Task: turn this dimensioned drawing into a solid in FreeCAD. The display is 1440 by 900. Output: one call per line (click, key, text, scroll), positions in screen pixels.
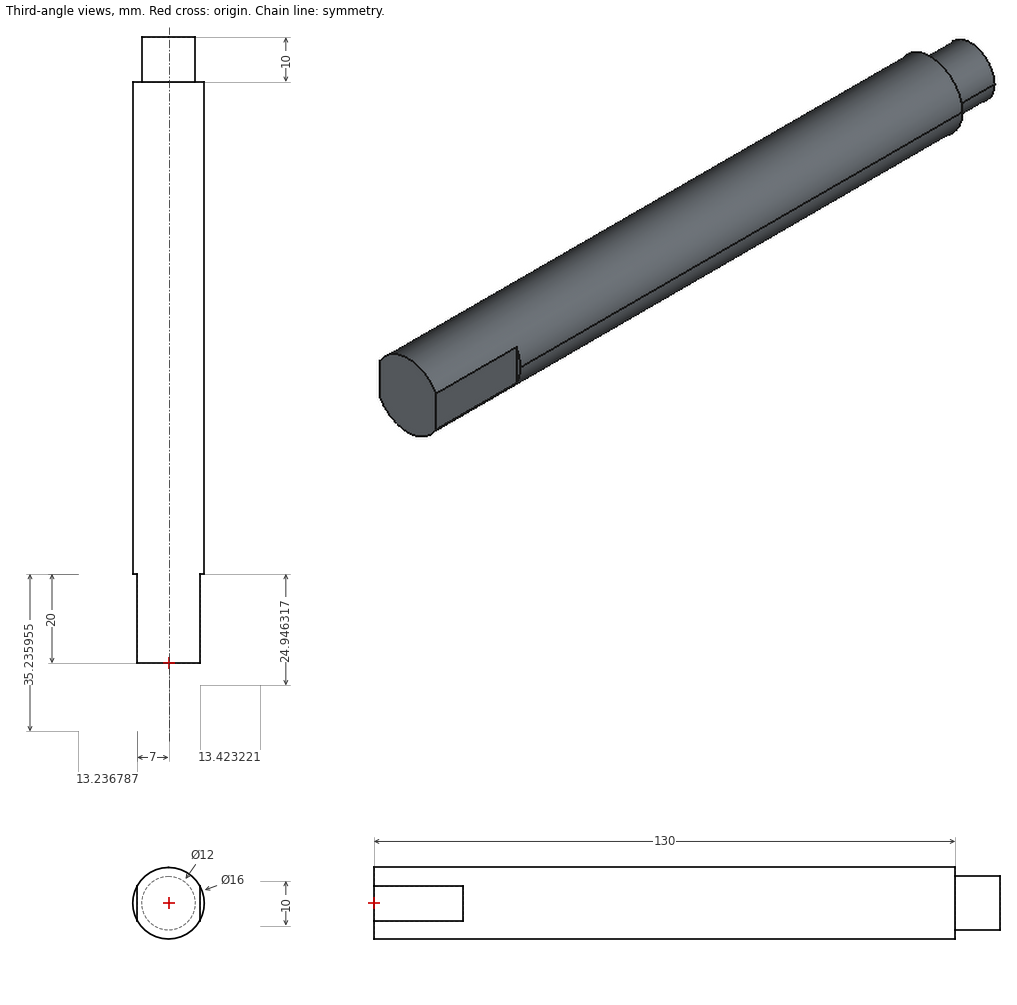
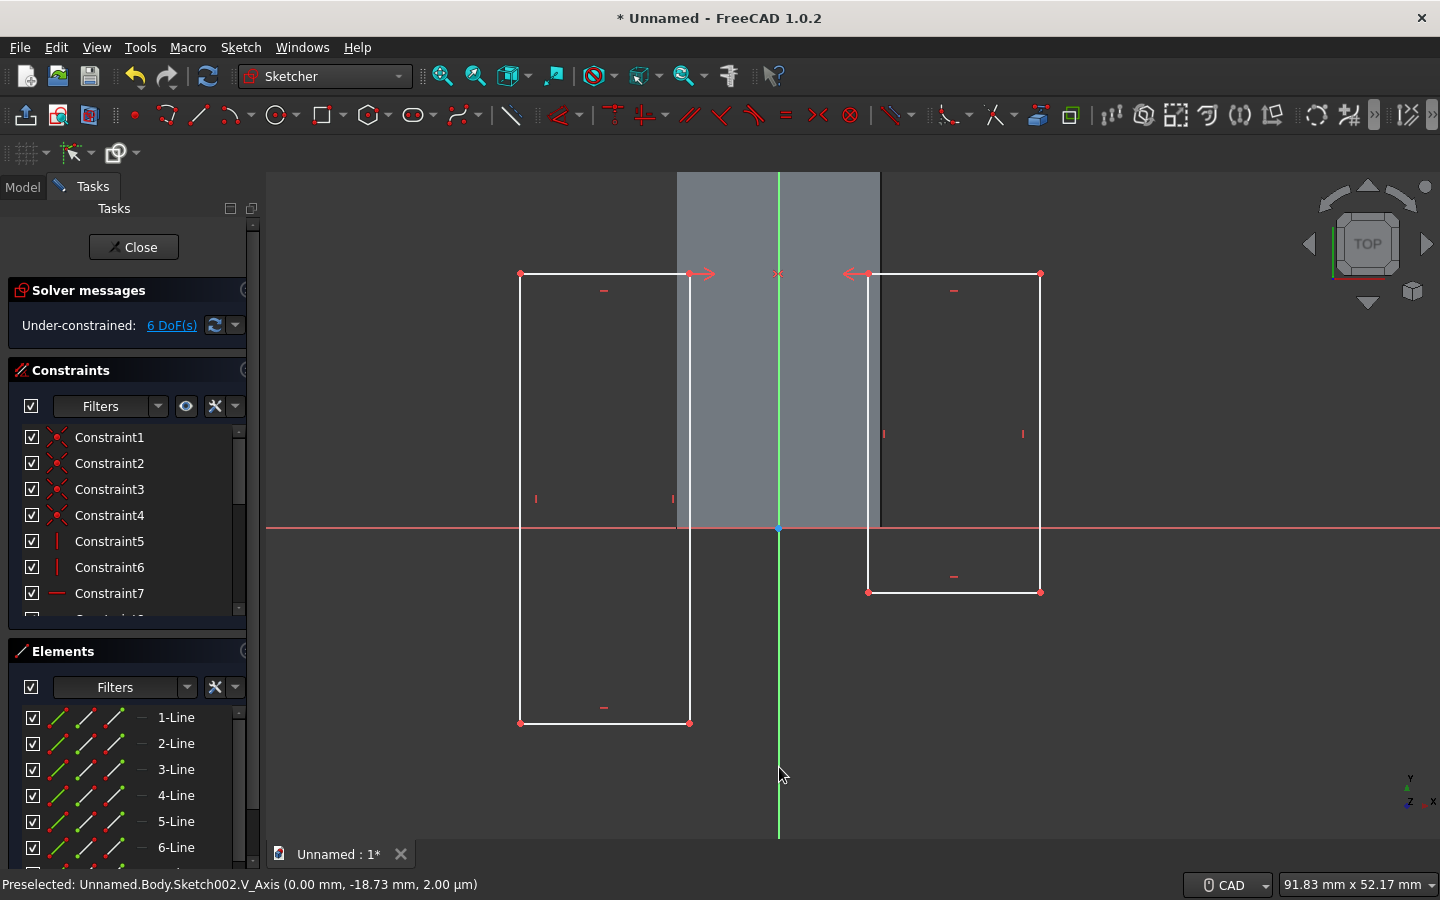
click(558, 116)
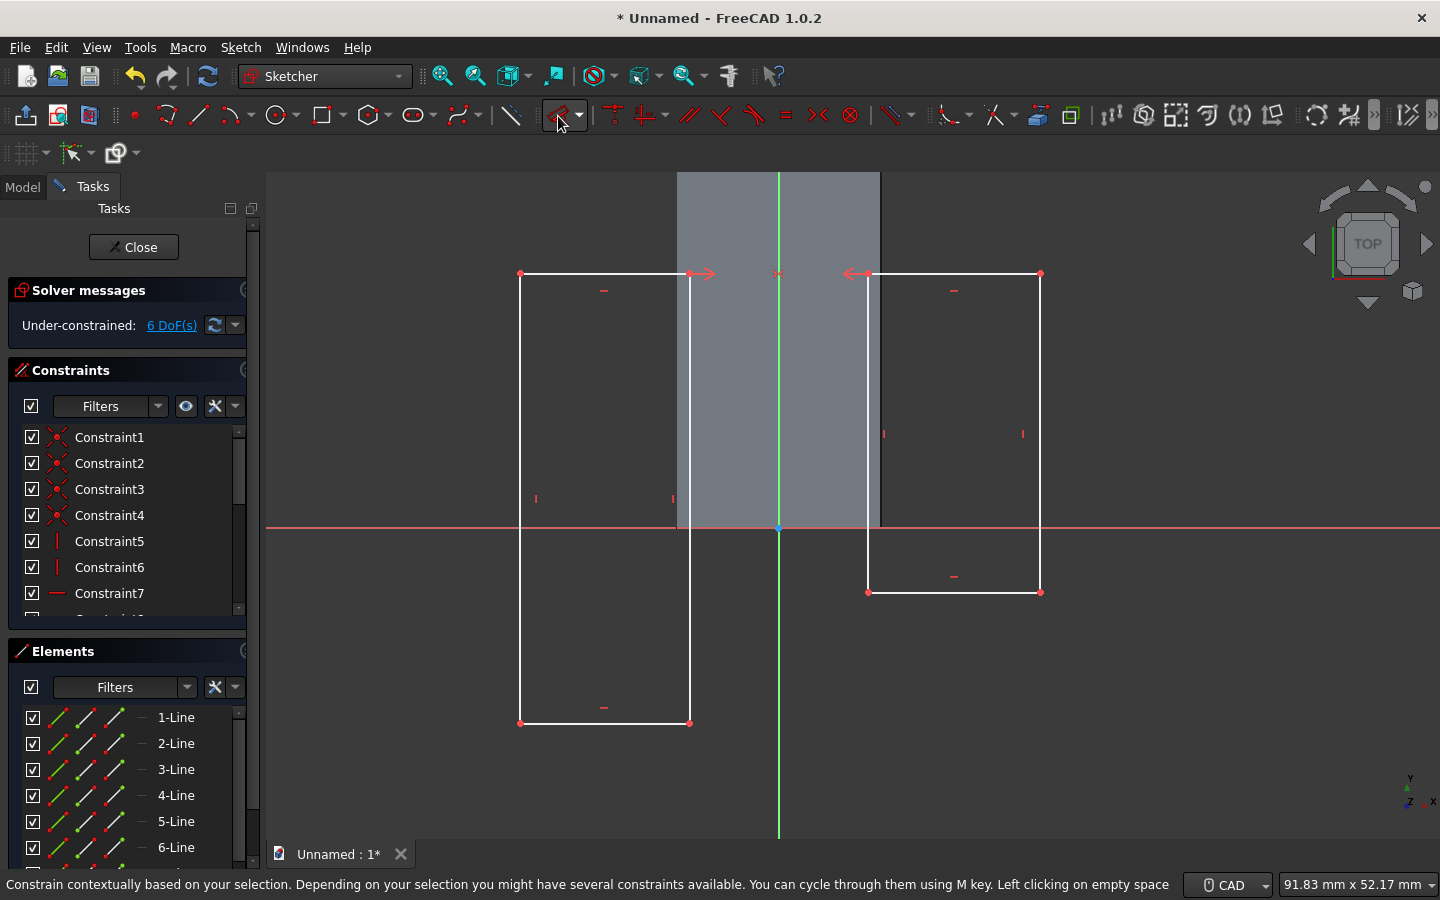
click(690, 724)
click(734, 758)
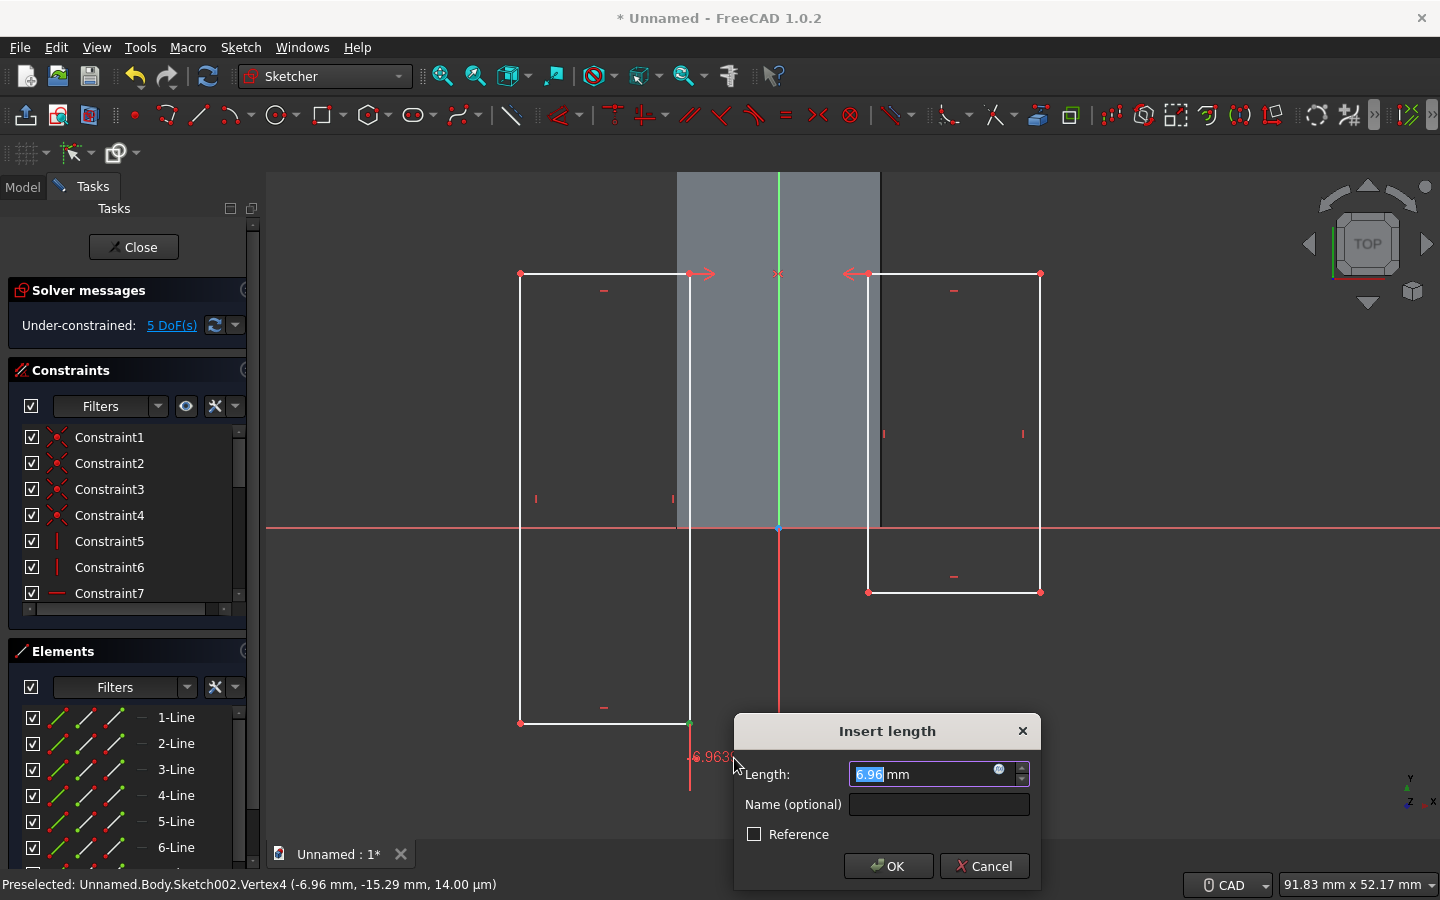
text(7)
key(Return)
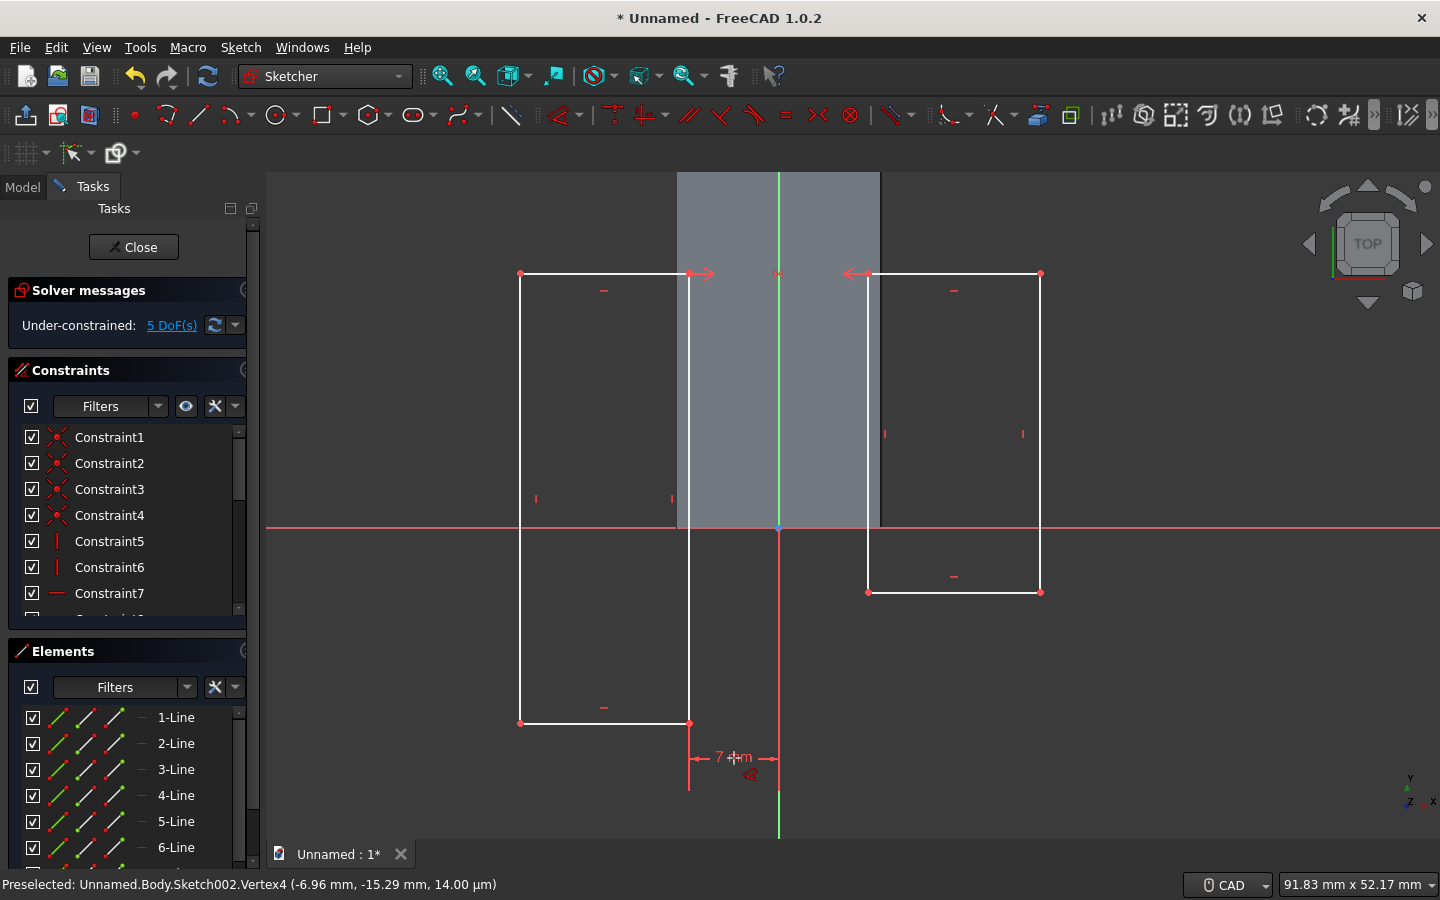
click(520, 274)
click(486, 401)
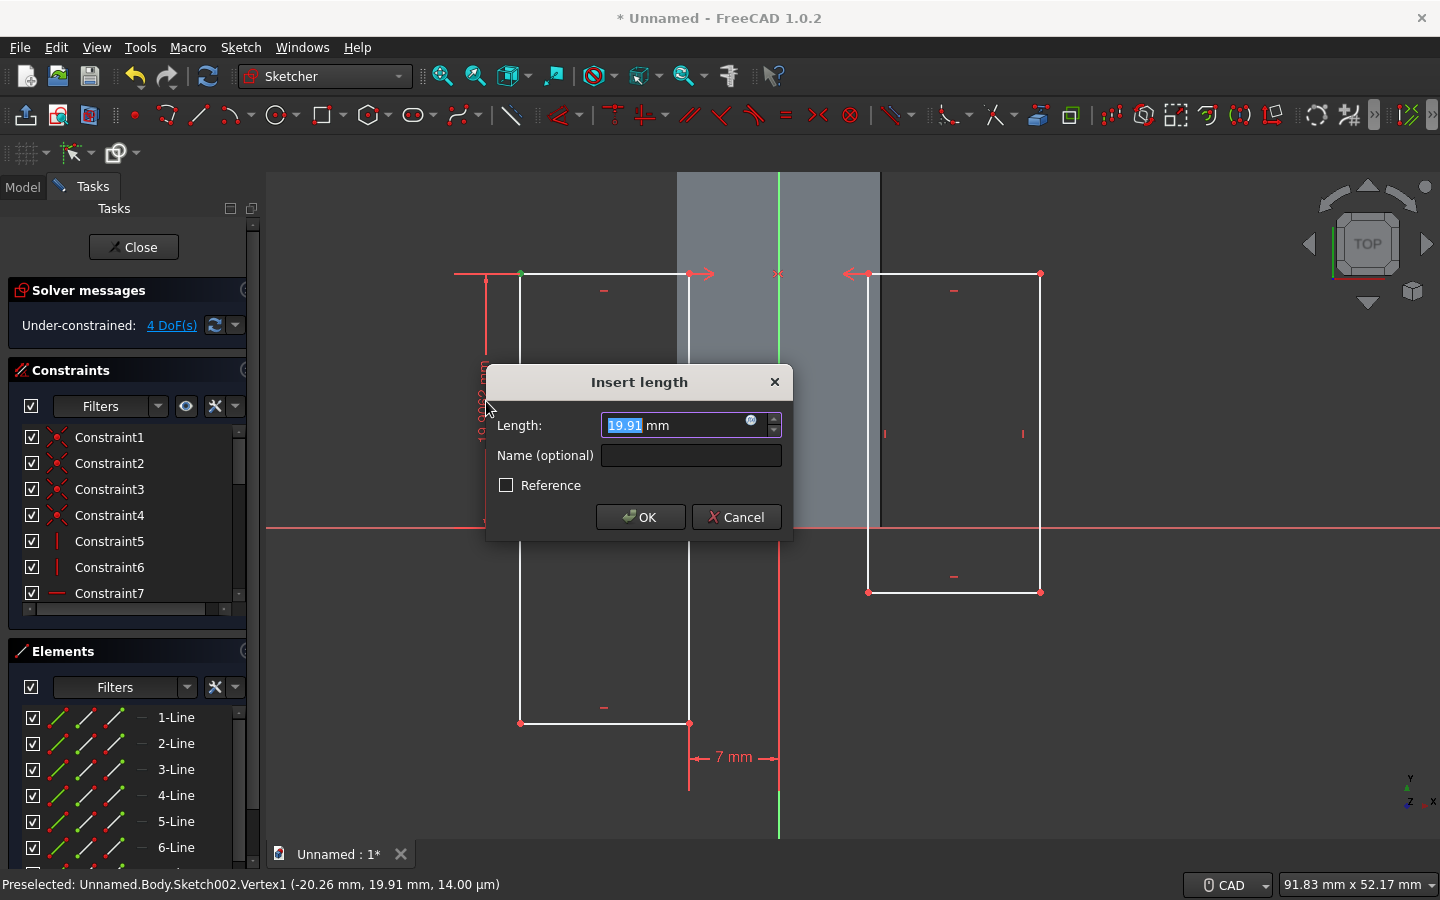
text(20)
key(Return)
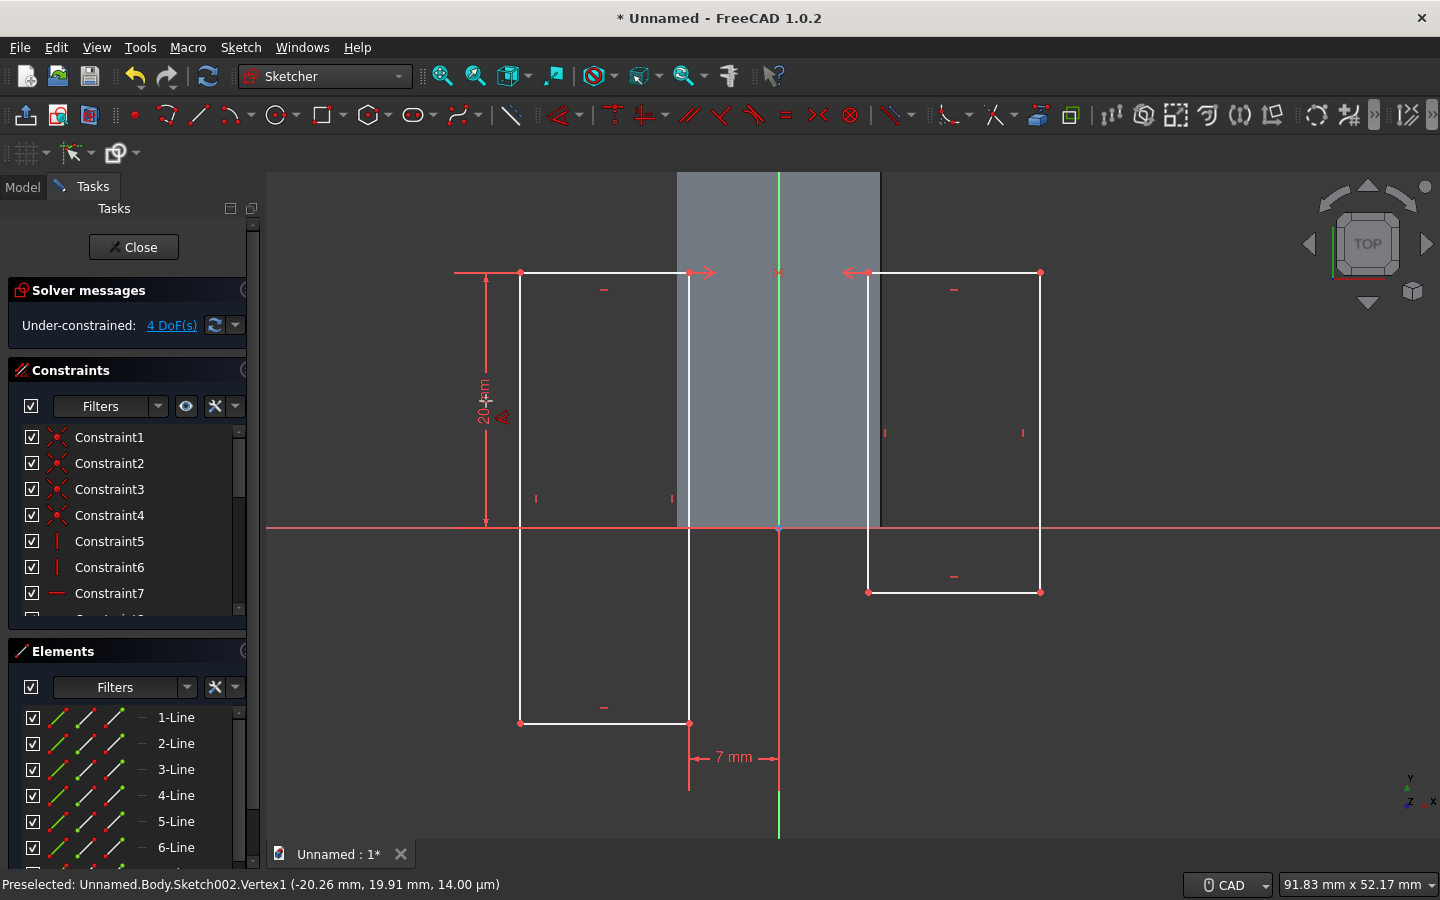
click(520, 408)
click(486, 498)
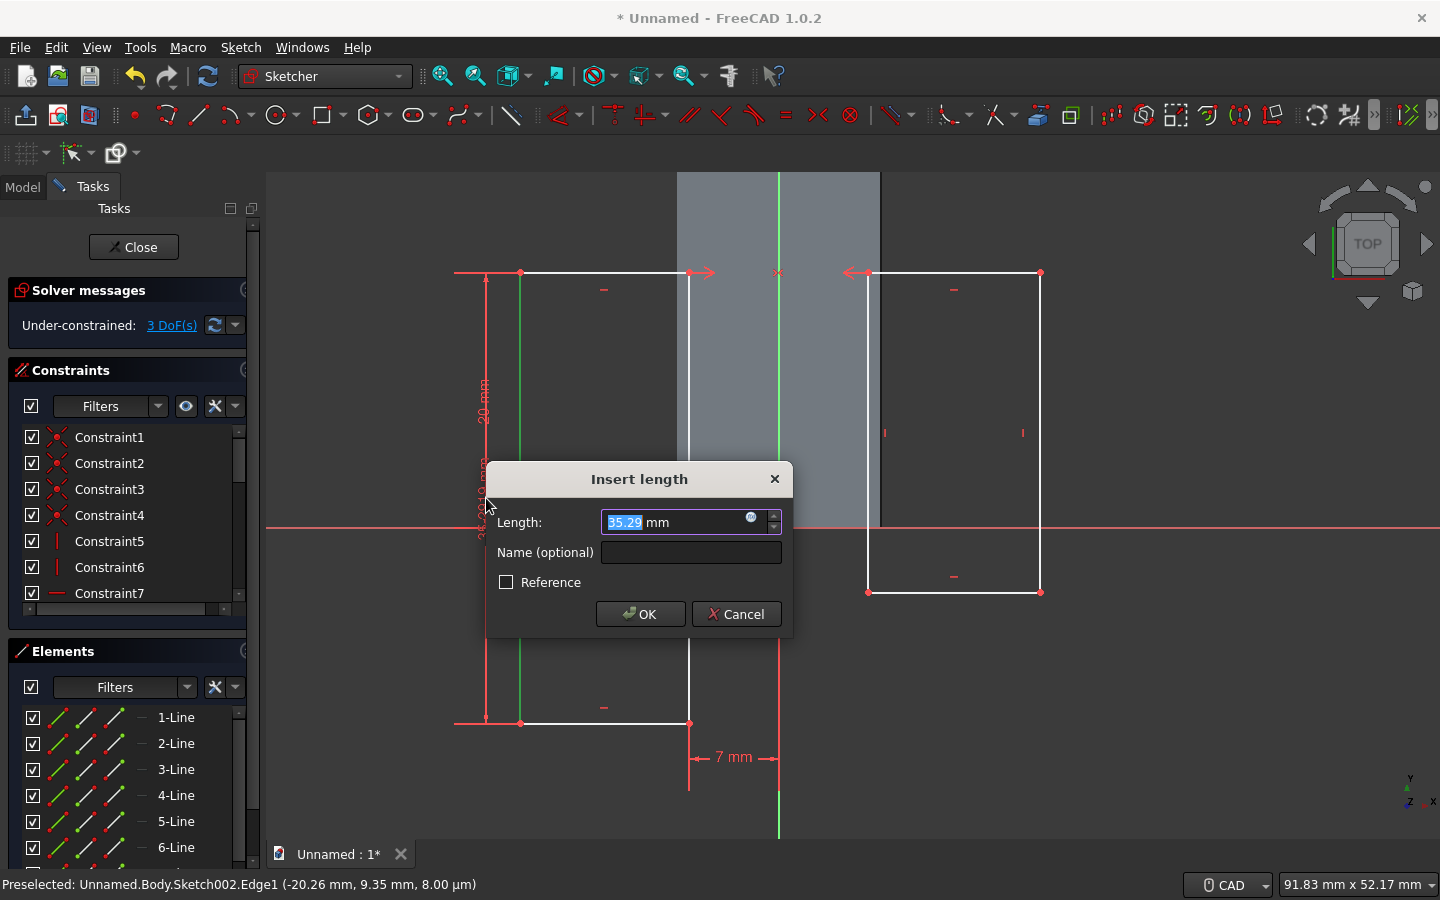
text(35.235955)
key(Return)